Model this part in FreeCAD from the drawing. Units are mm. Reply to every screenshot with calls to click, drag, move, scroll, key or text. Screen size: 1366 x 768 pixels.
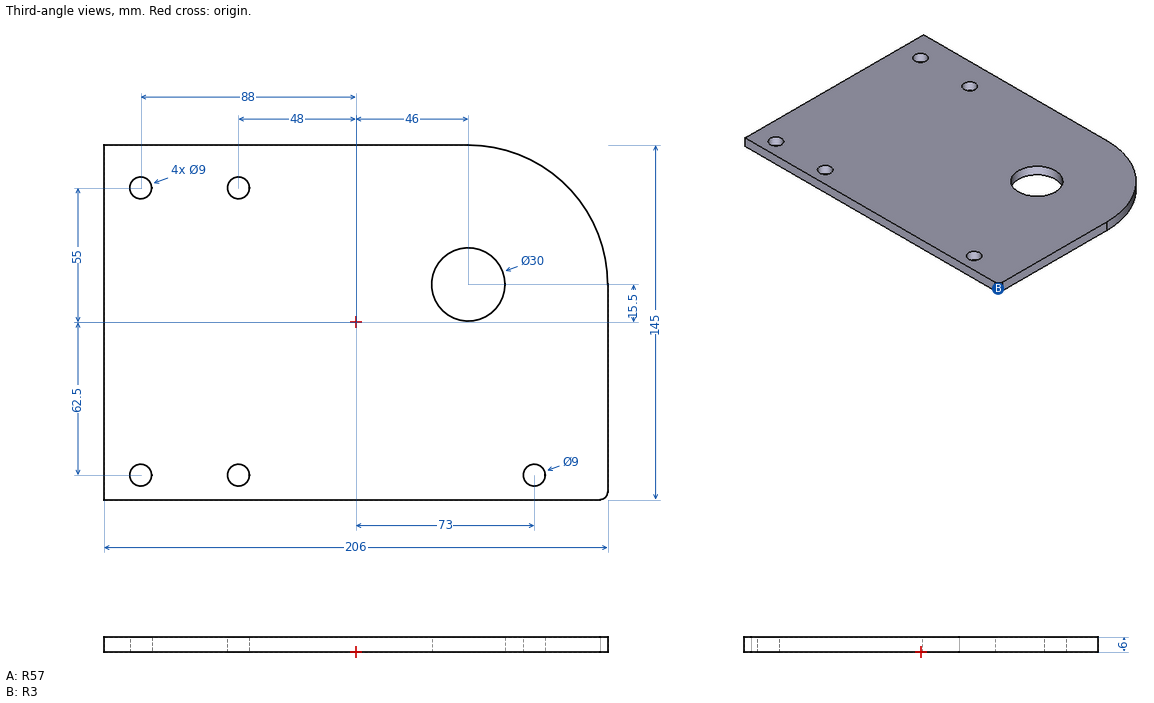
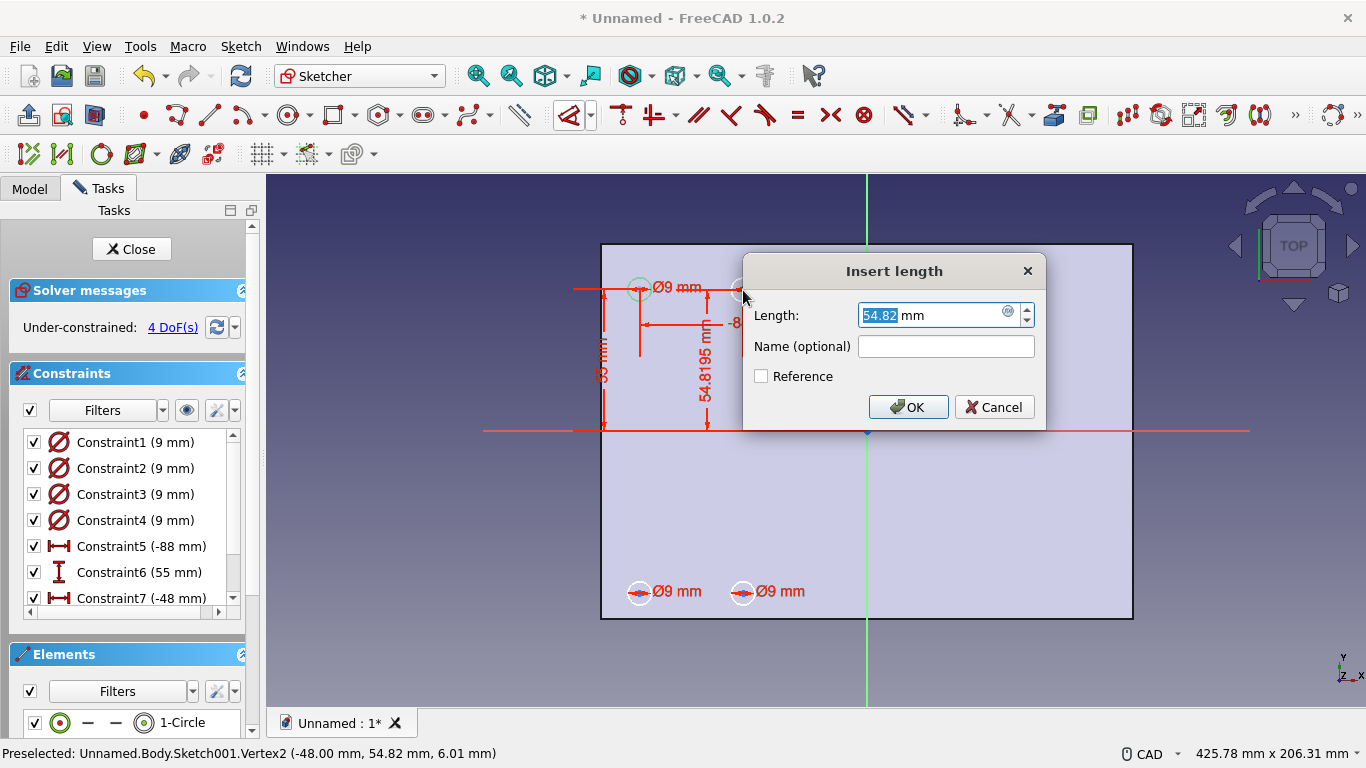
text(55)
key(Return)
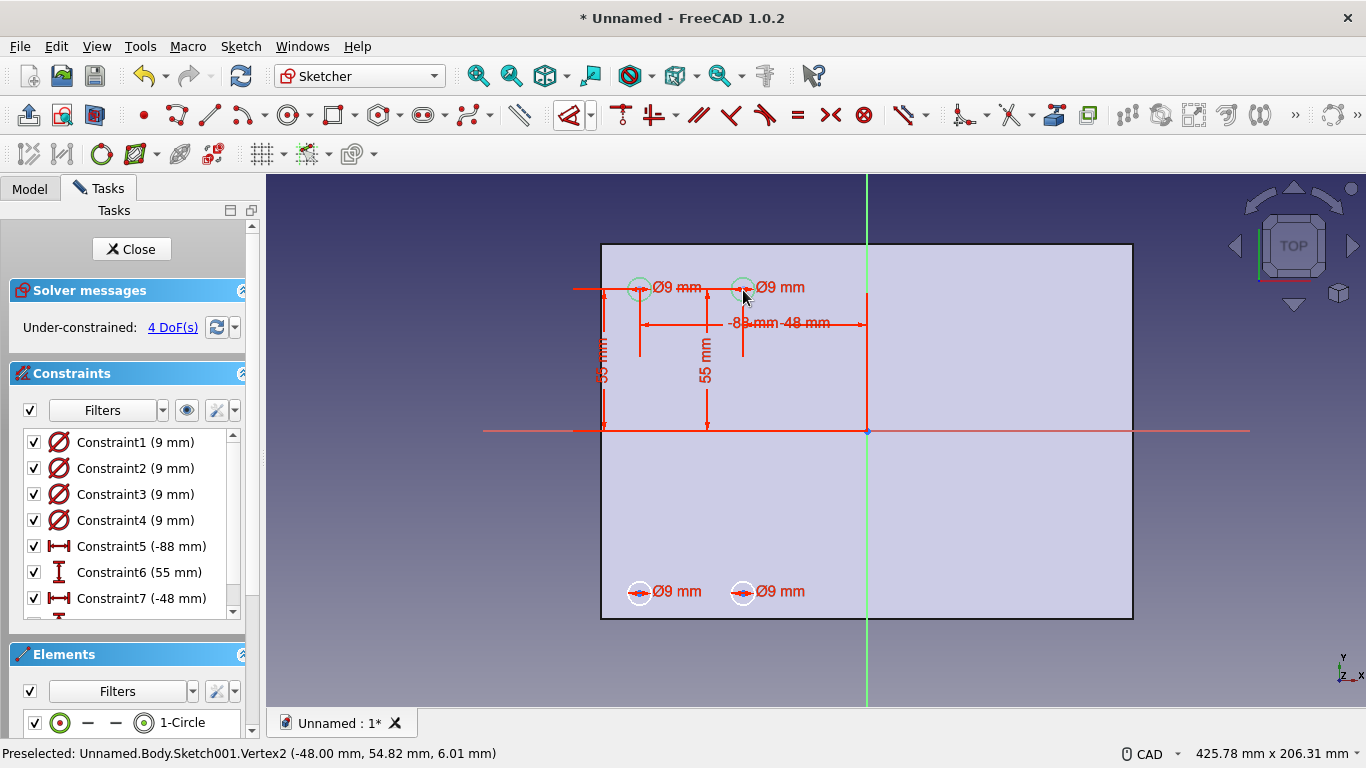
click(640, 593)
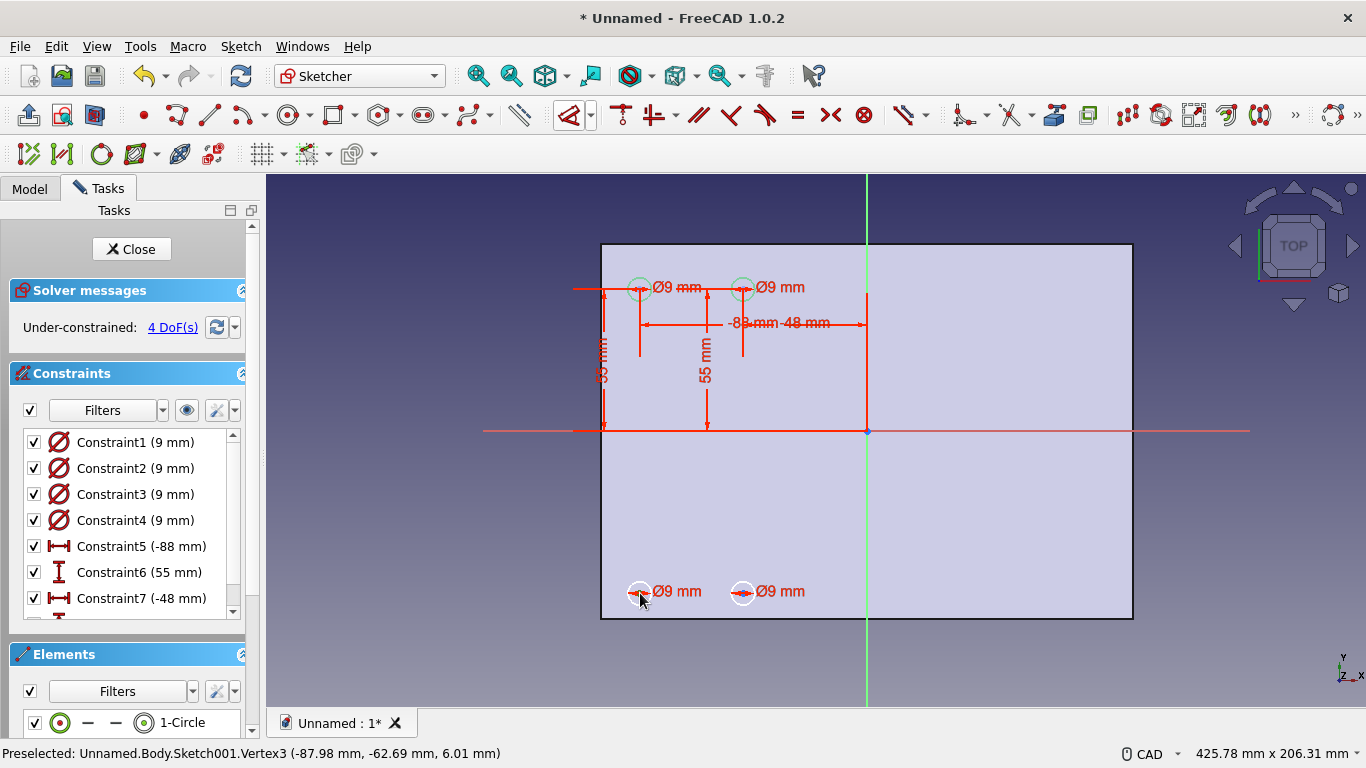
key(l)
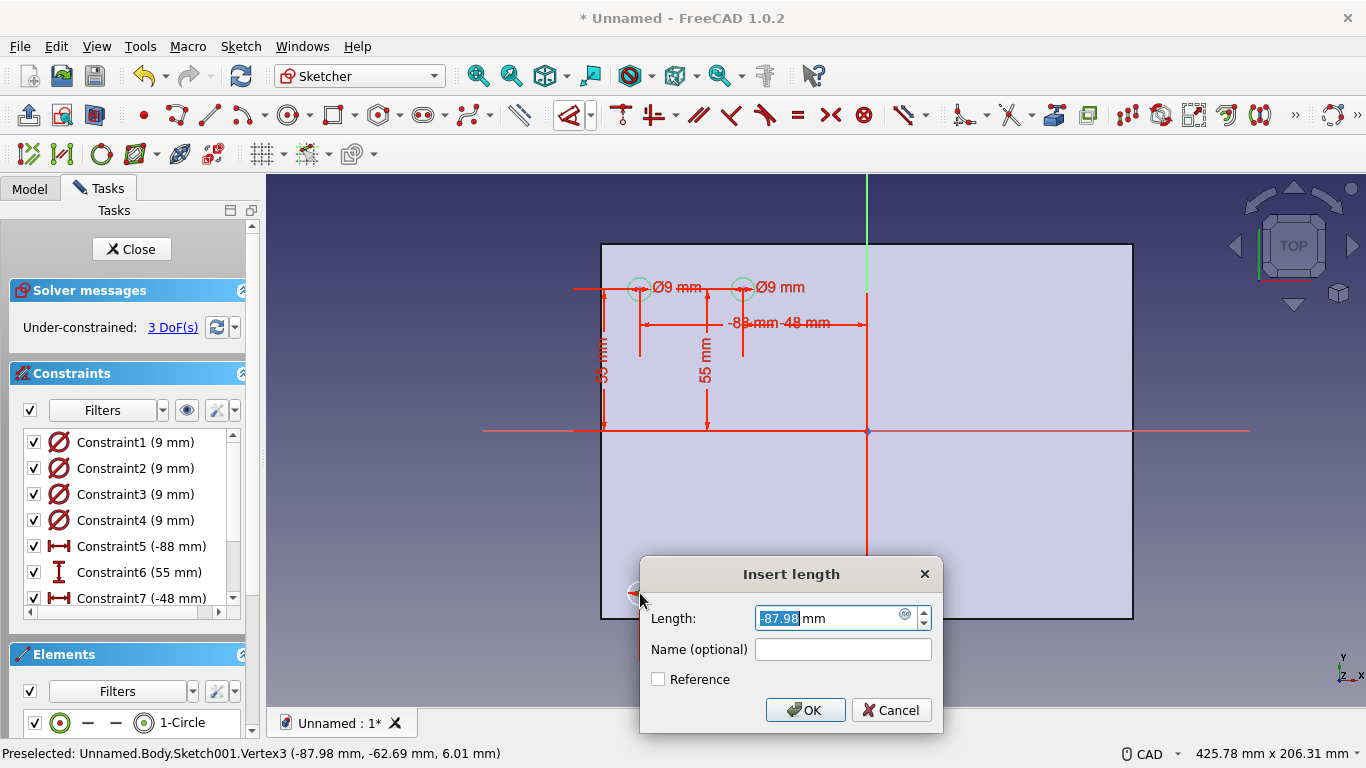
text(-88)
key(Return)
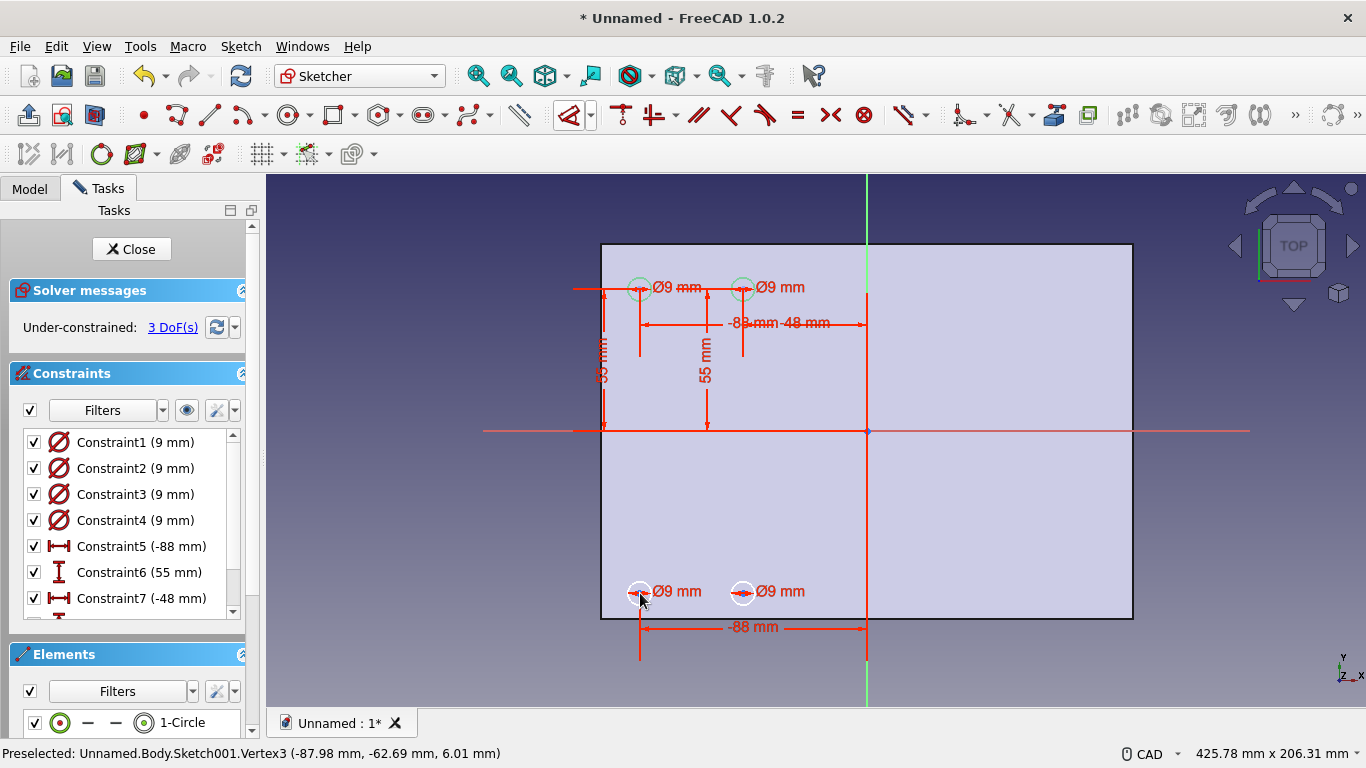
click(743, 593)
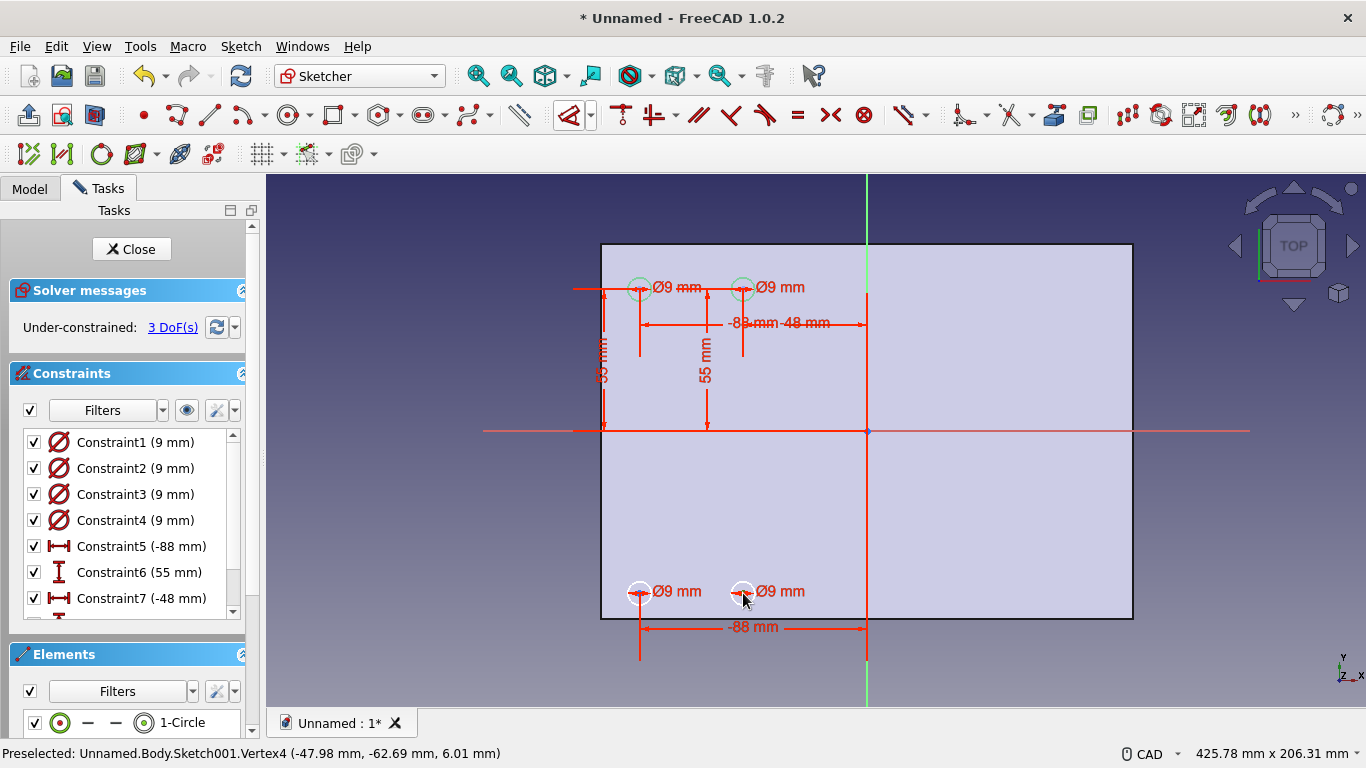
click(590, 116)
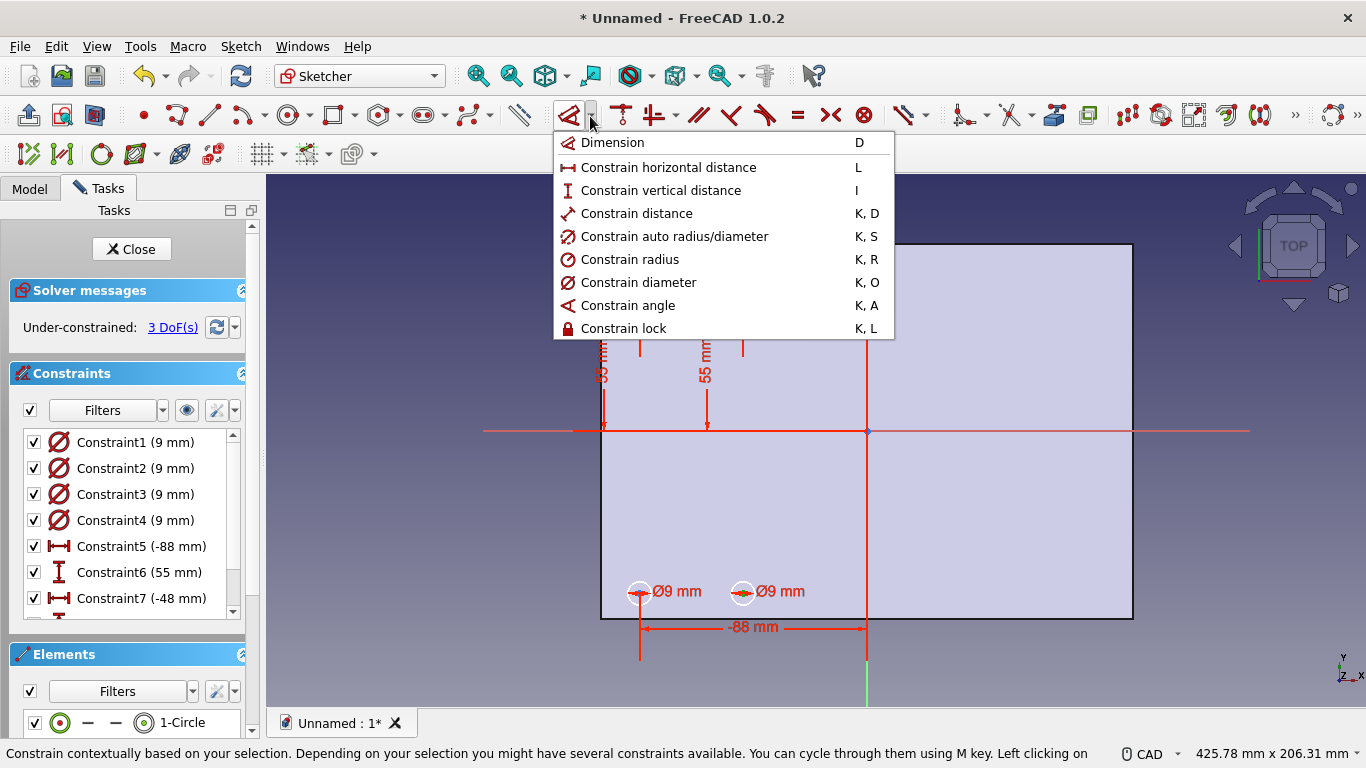
click(724, 168)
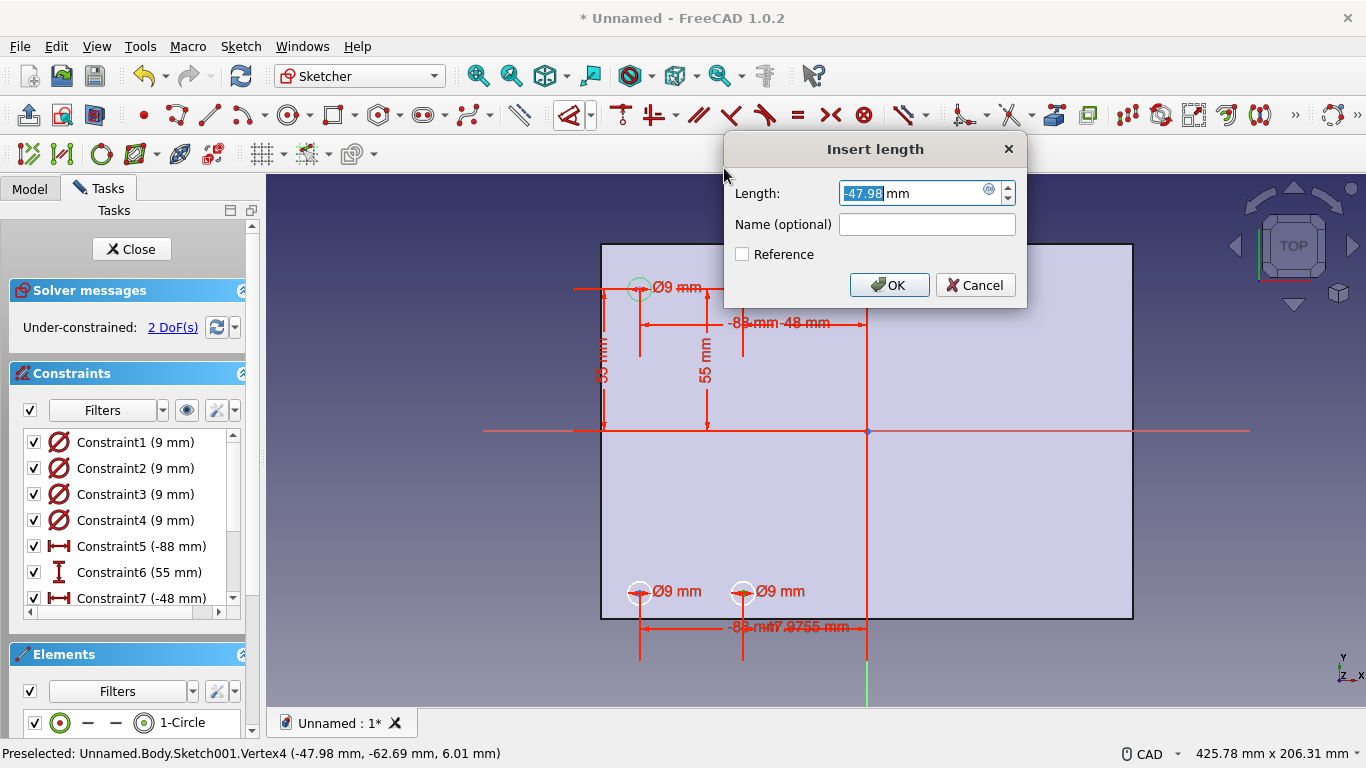
text(-48)
key(Return)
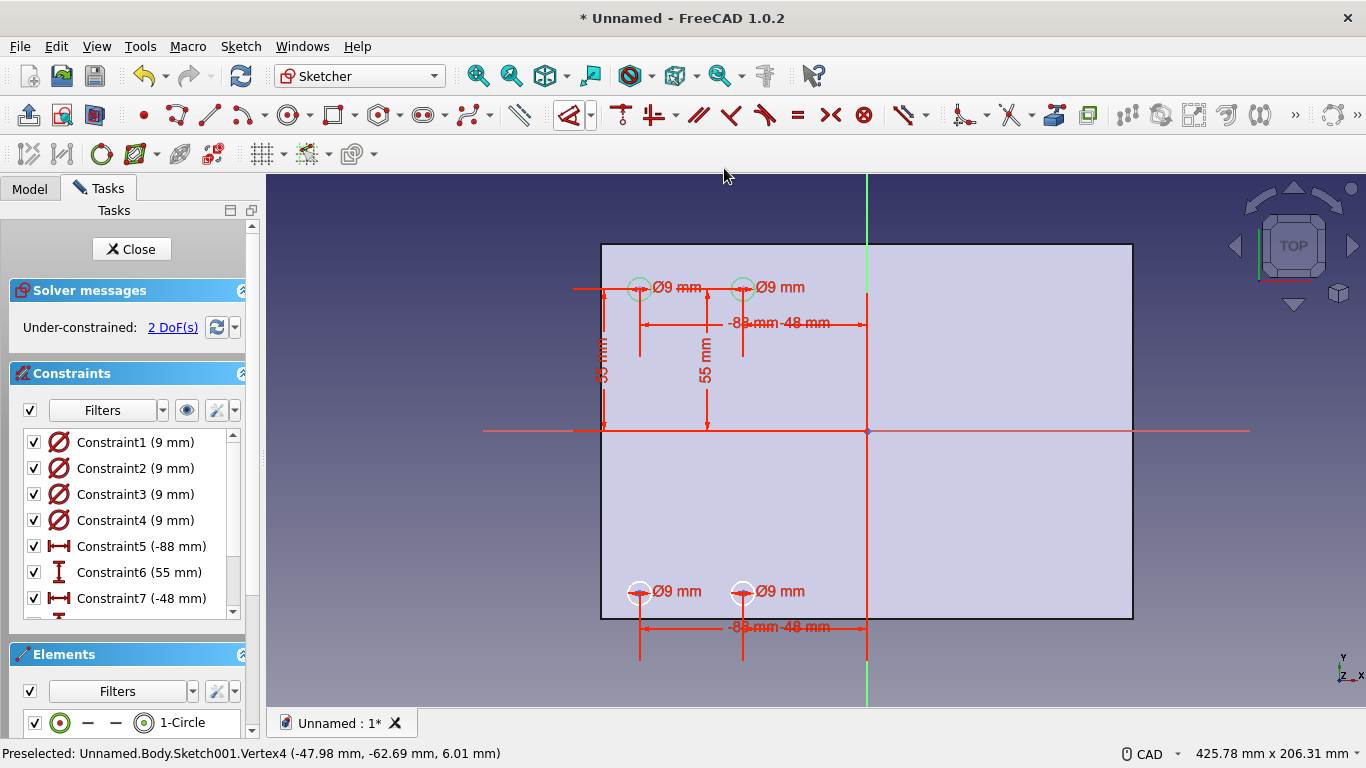
click(640, 593)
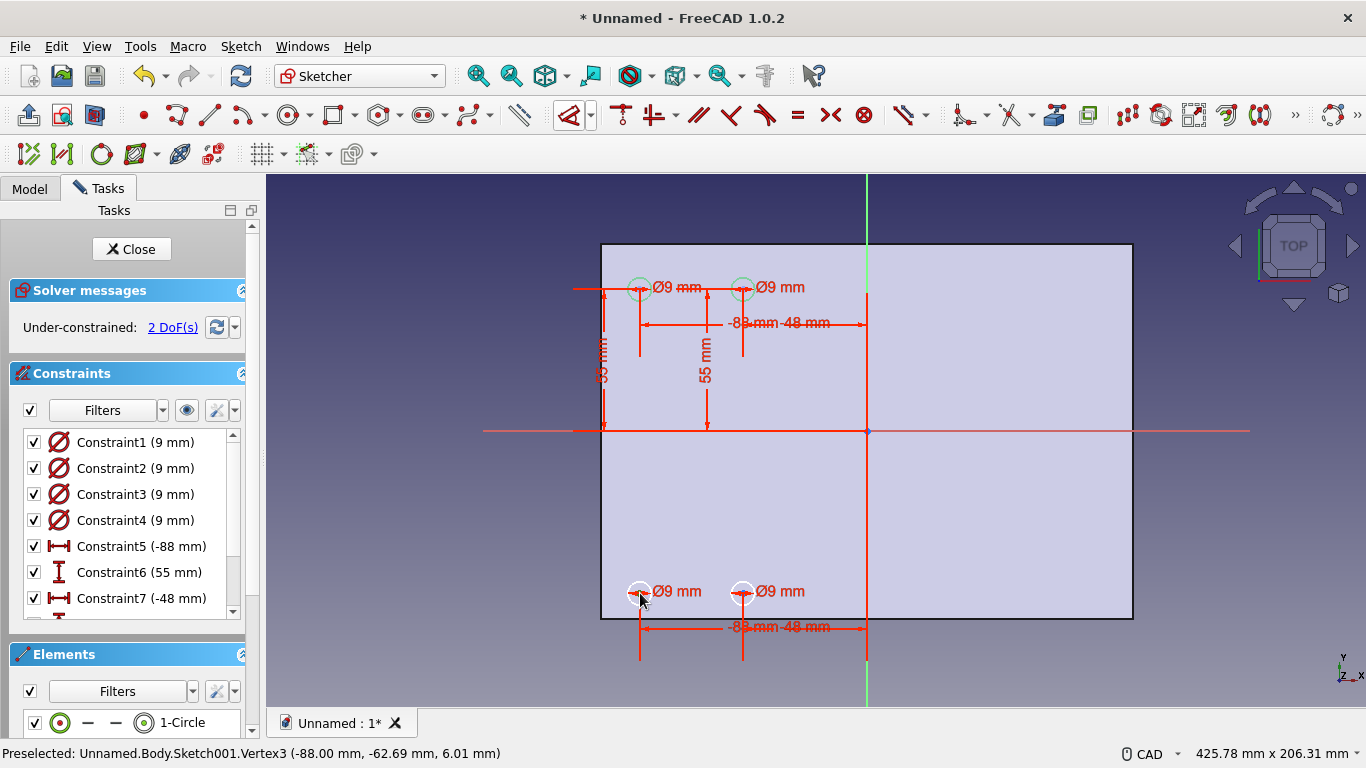
key(i)